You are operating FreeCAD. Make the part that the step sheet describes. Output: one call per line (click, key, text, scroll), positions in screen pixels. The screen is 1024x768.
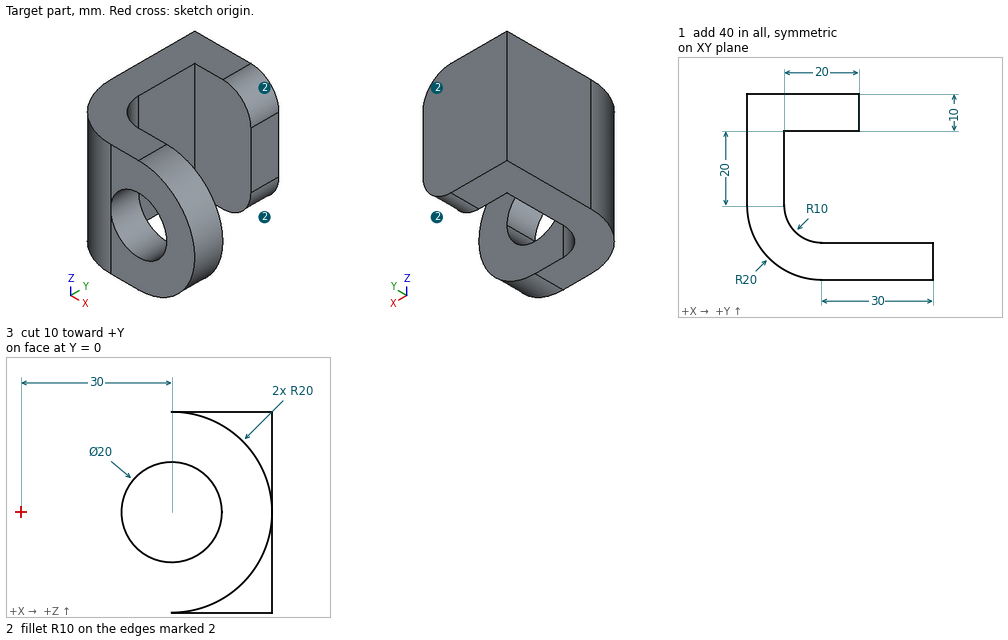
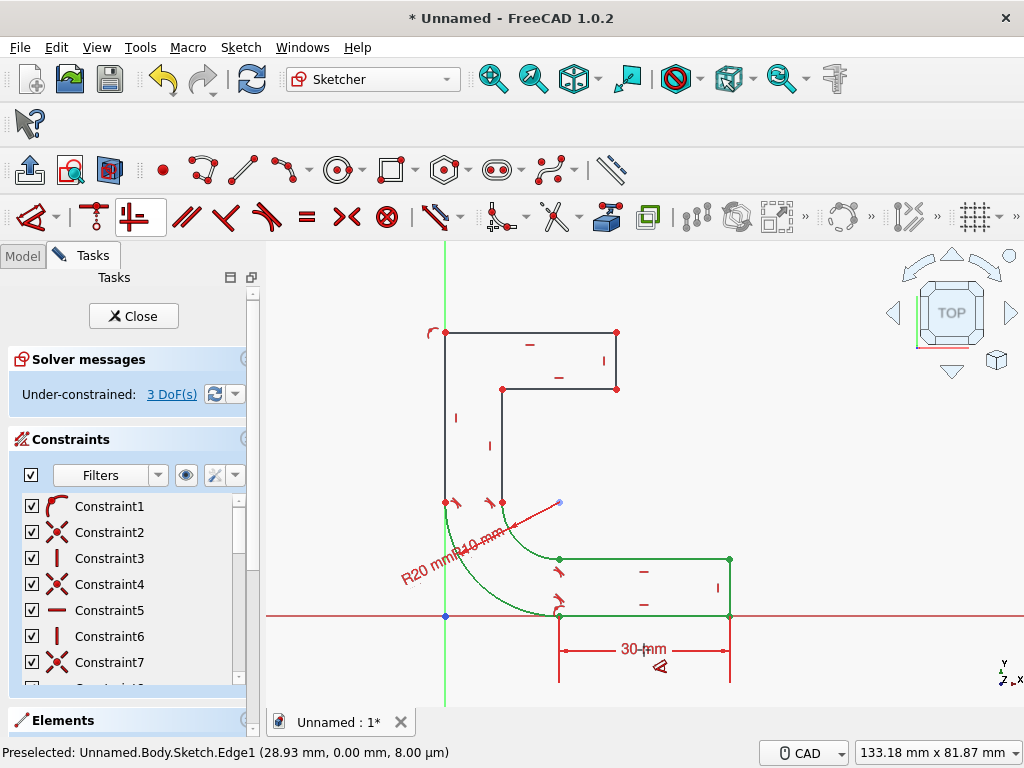
click(502, 469)
click(468, 446)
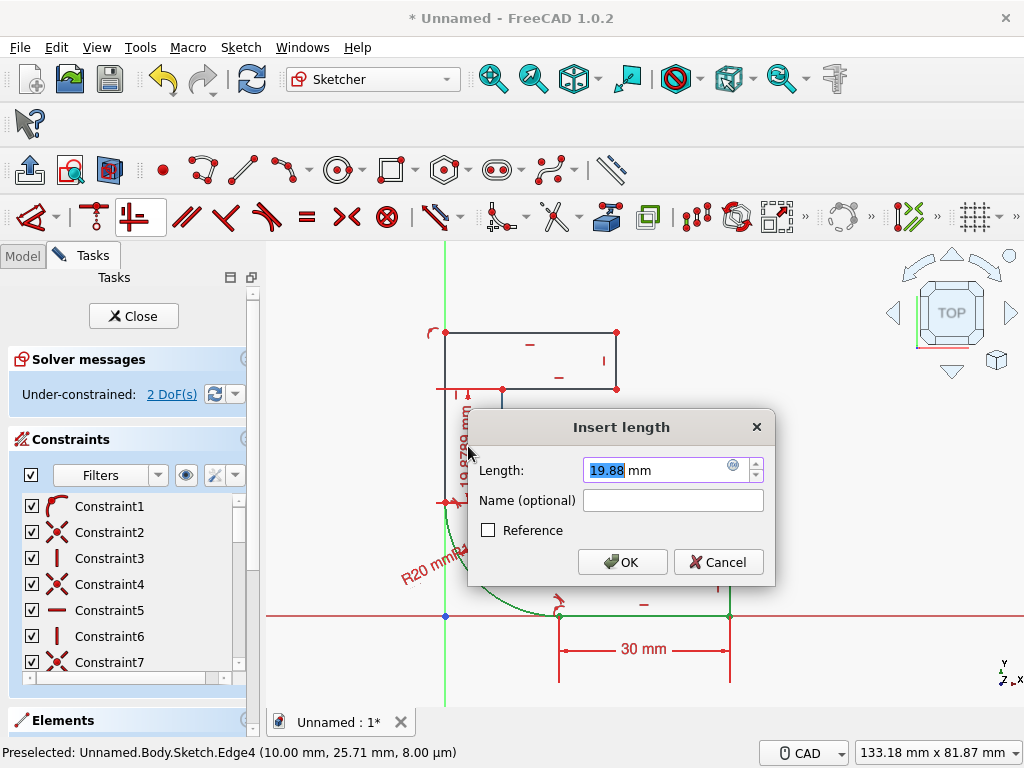
text(20)
key(Return)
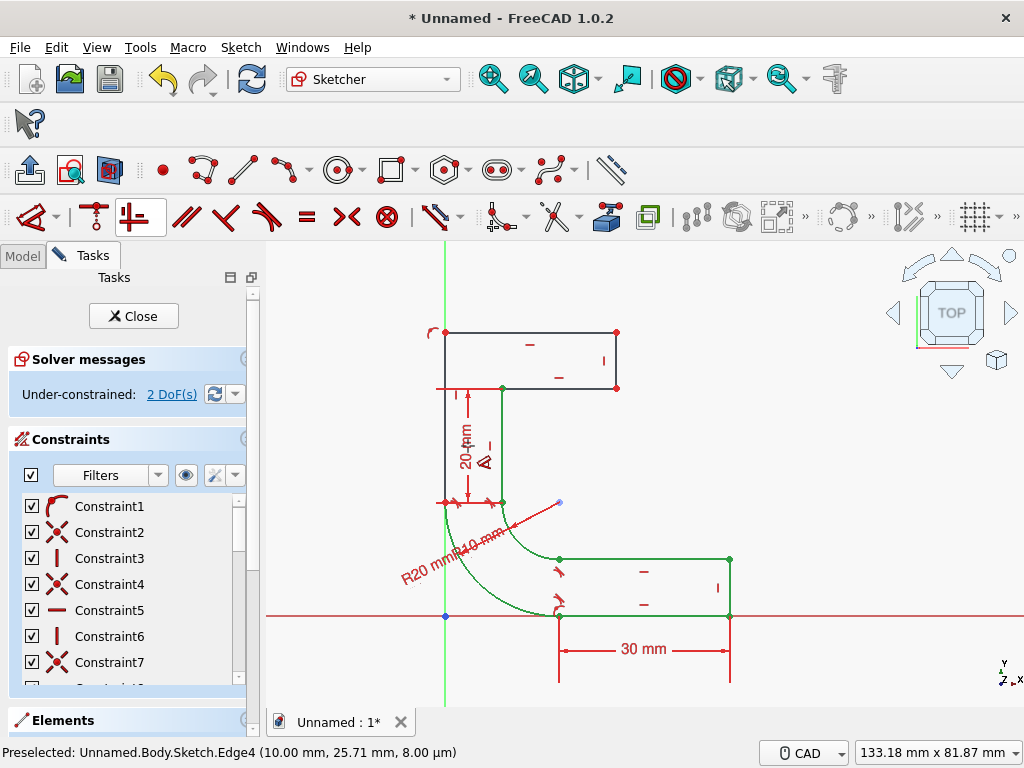
click(536, 389)
click(559, 355)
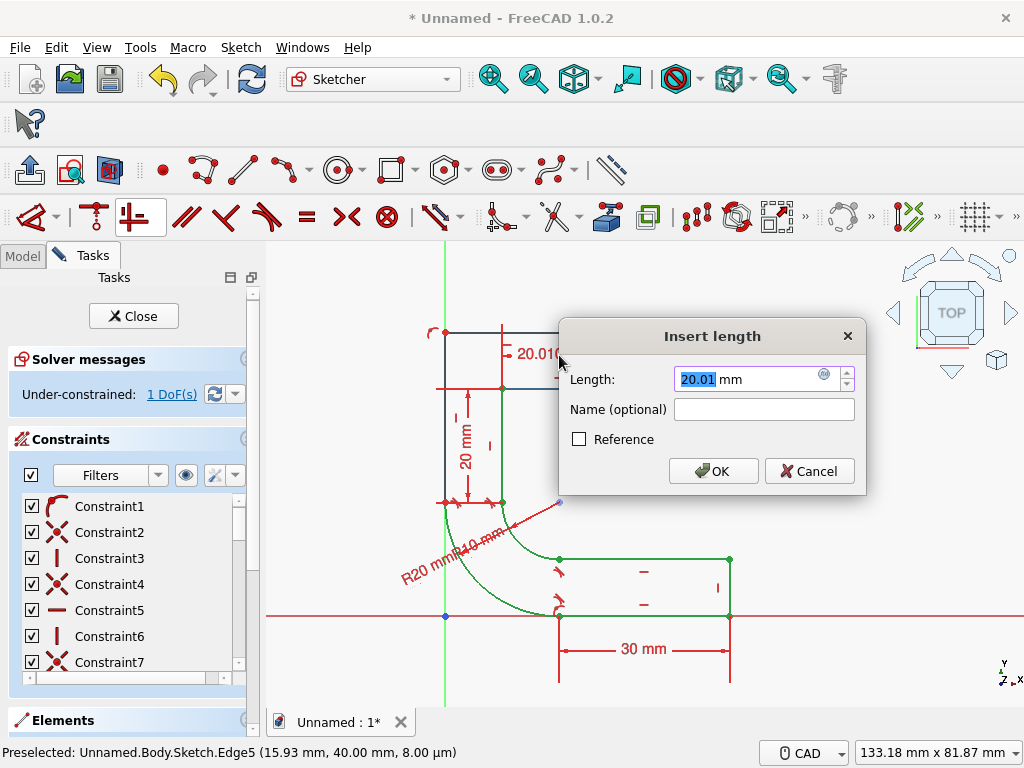
text(20)
key(Return)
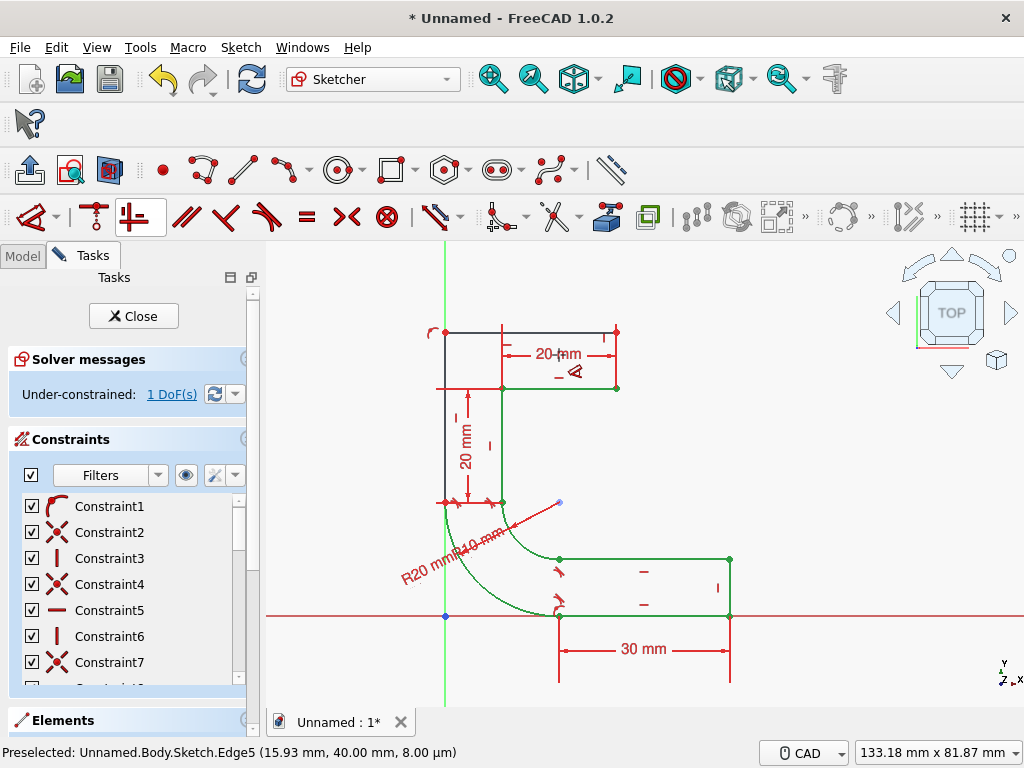
click(616, 372)
click(650, 361)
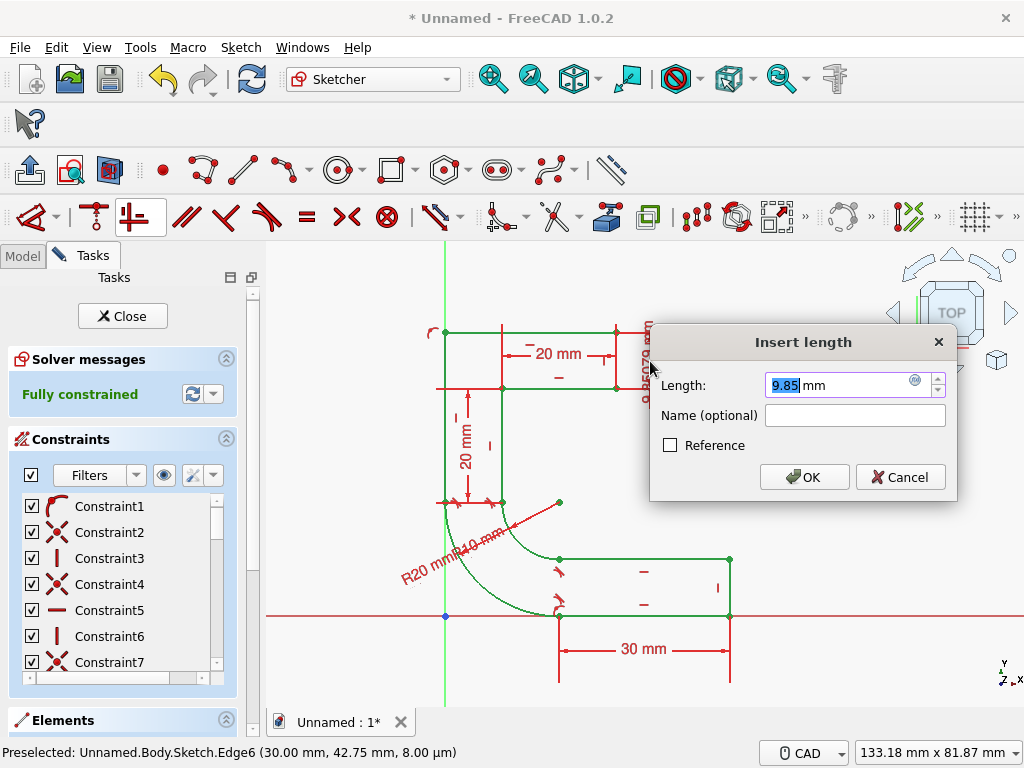
text(10)
key(Return)
key(Escape)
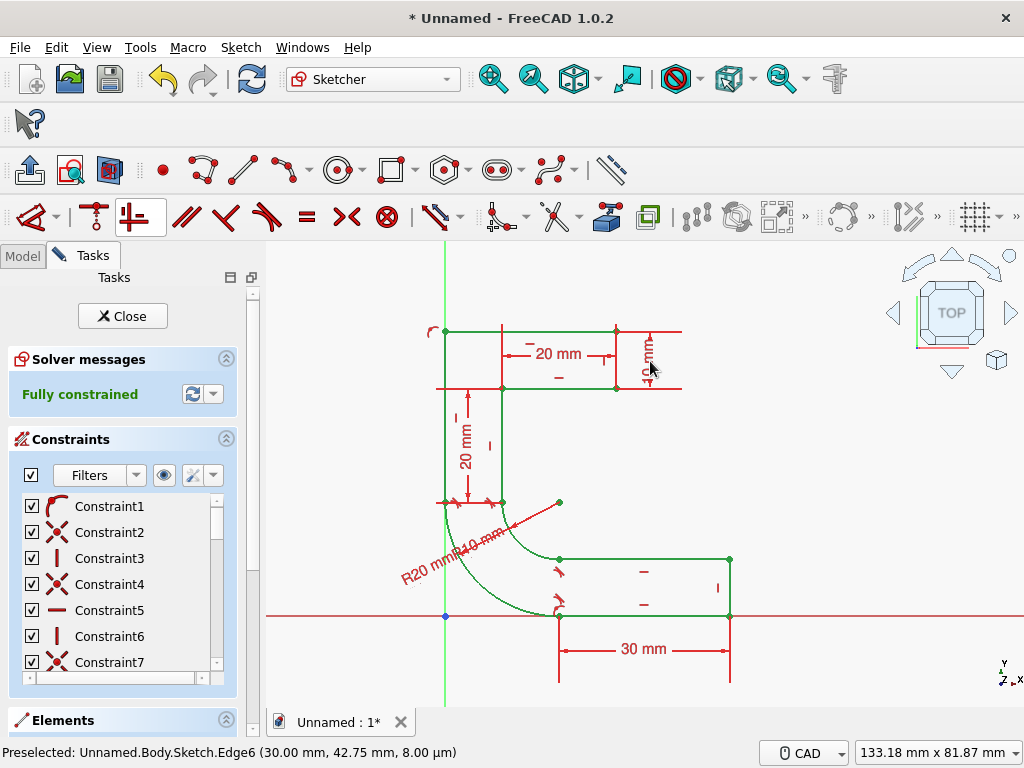
click(123, 316)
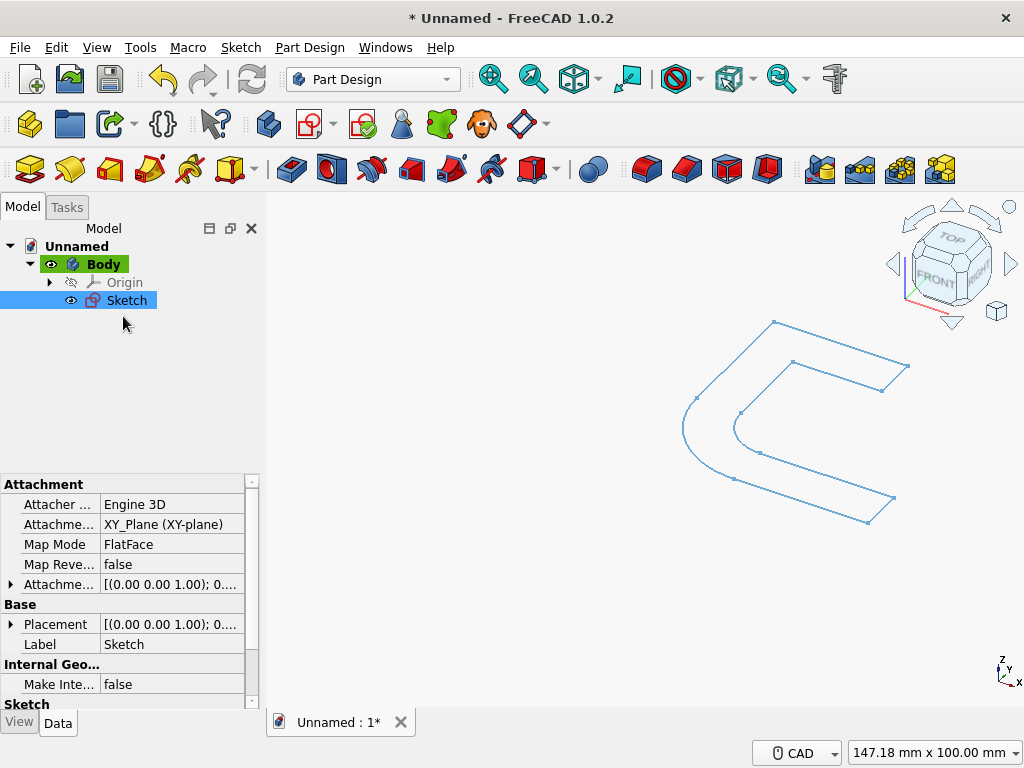
click(30, 170)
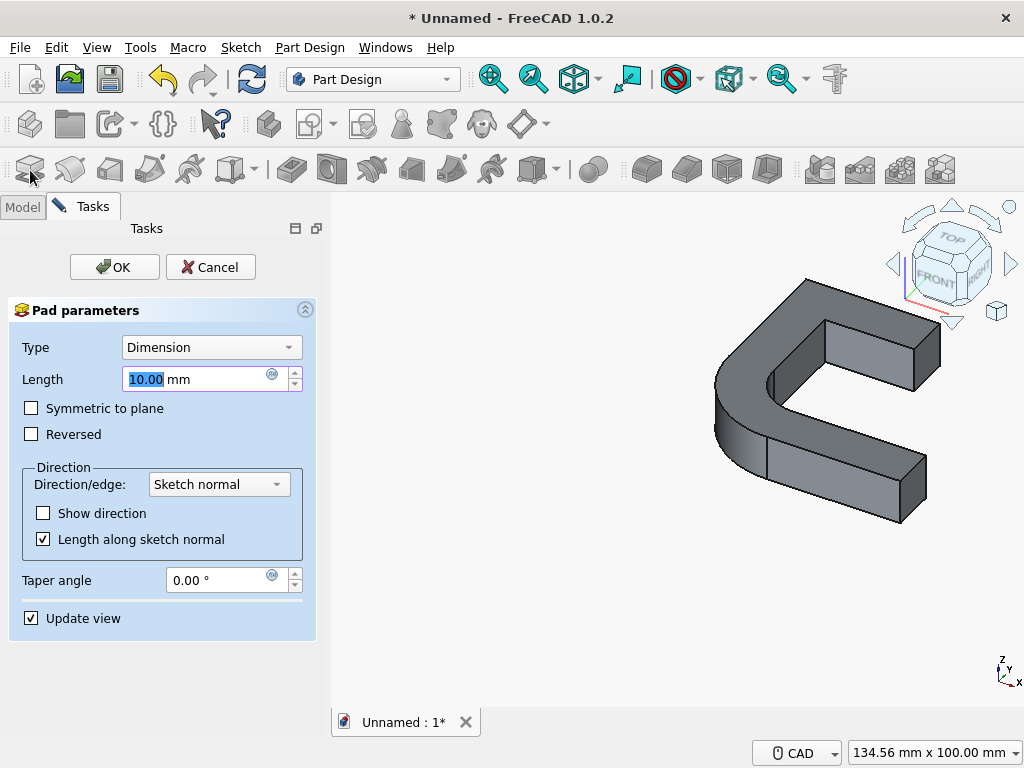
text(40)
key(Tab)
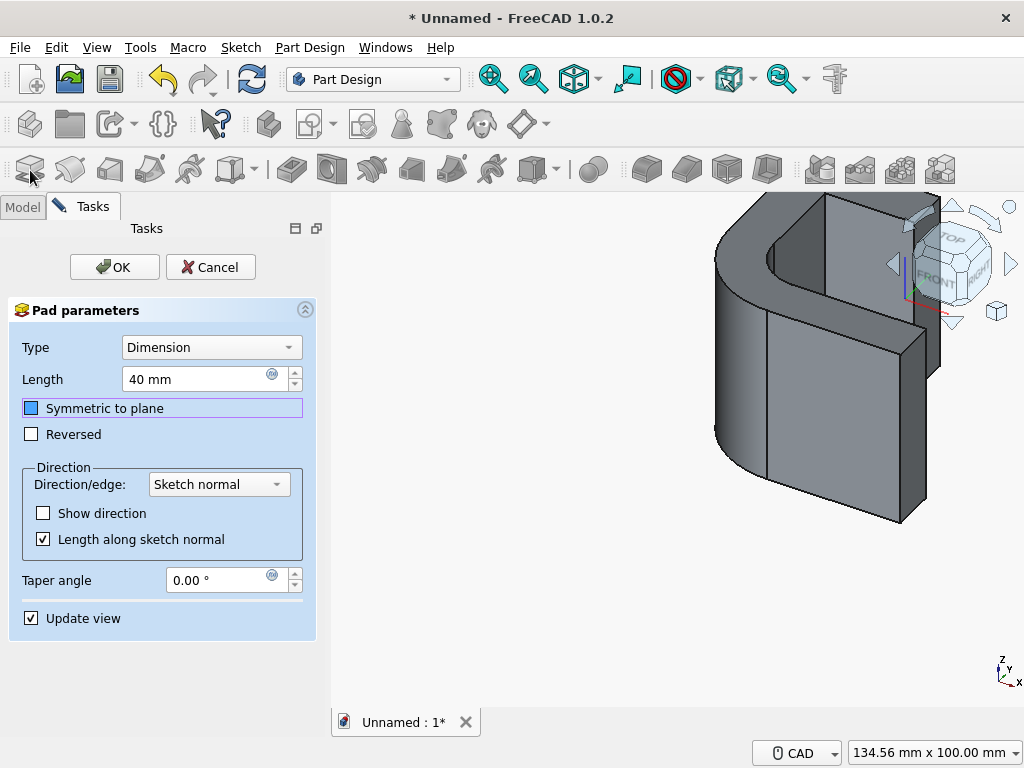
click(30, 408)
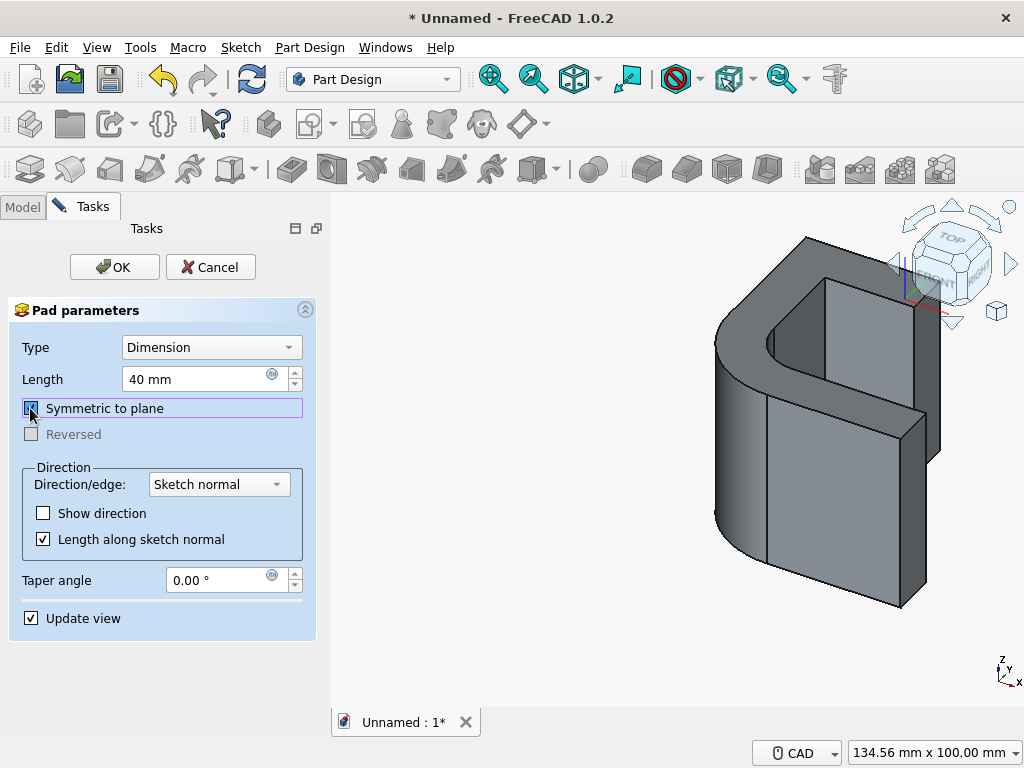
click(115, 267)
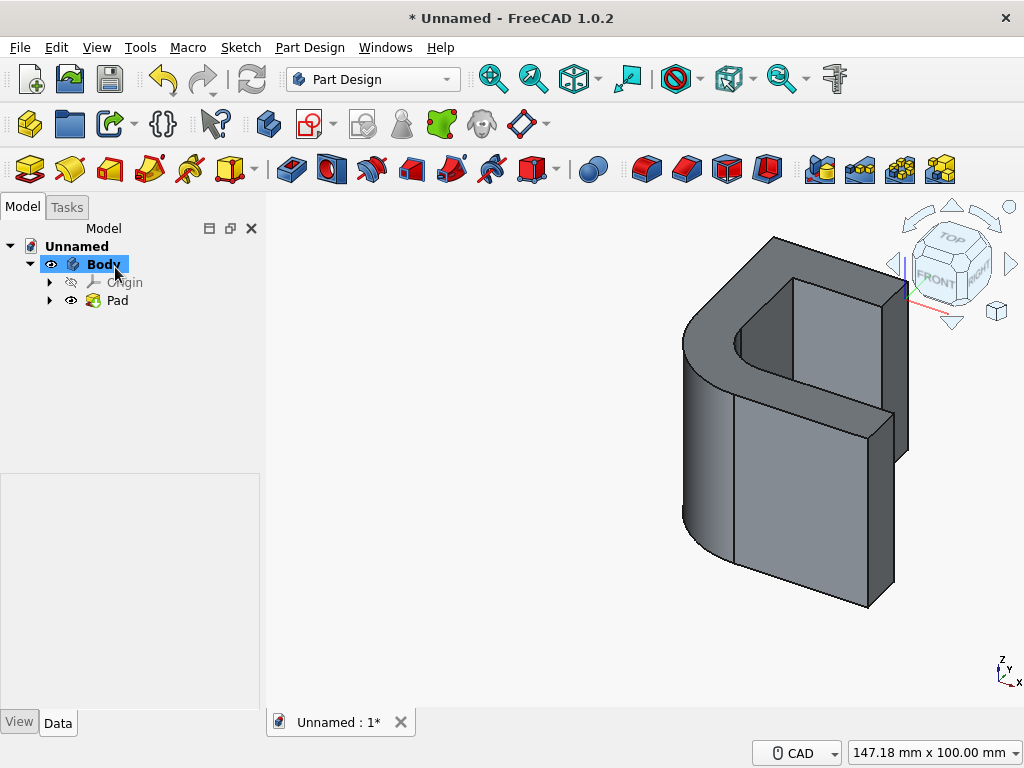
key(0)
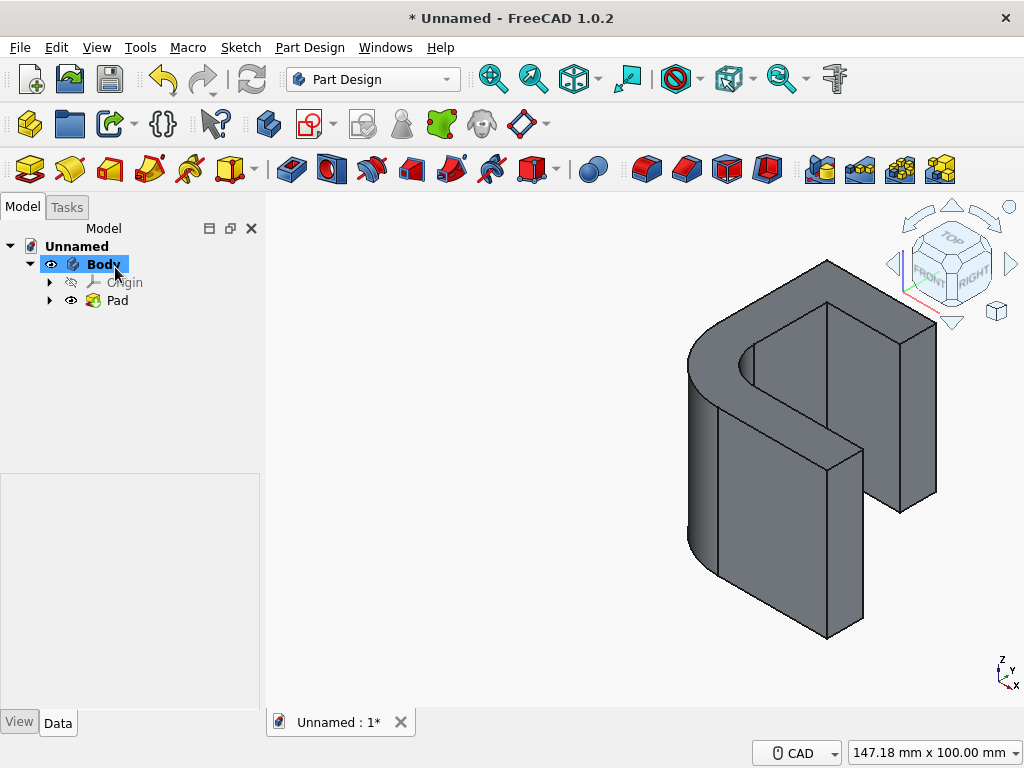
key(2)